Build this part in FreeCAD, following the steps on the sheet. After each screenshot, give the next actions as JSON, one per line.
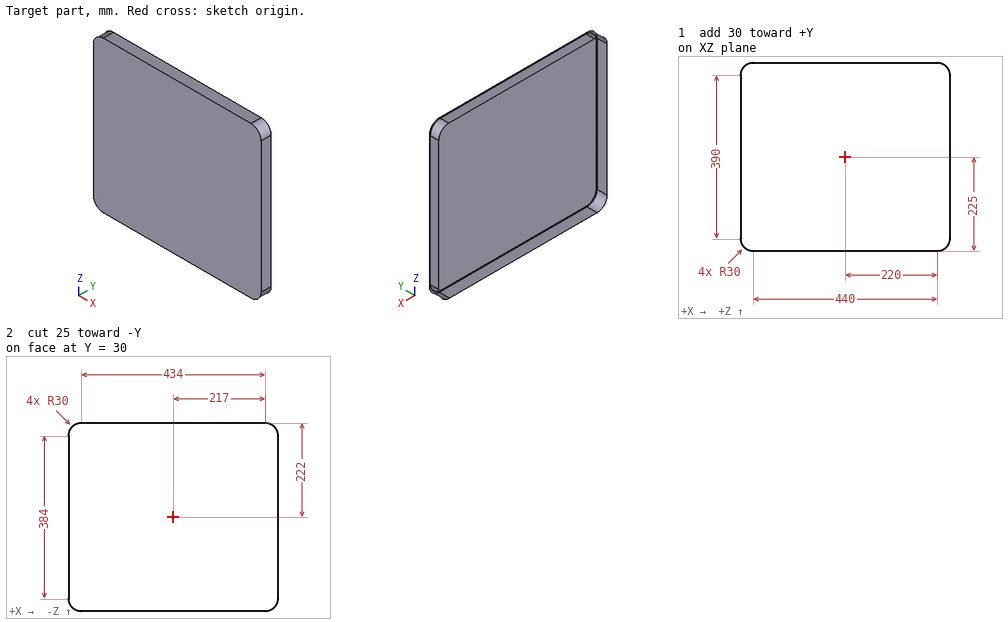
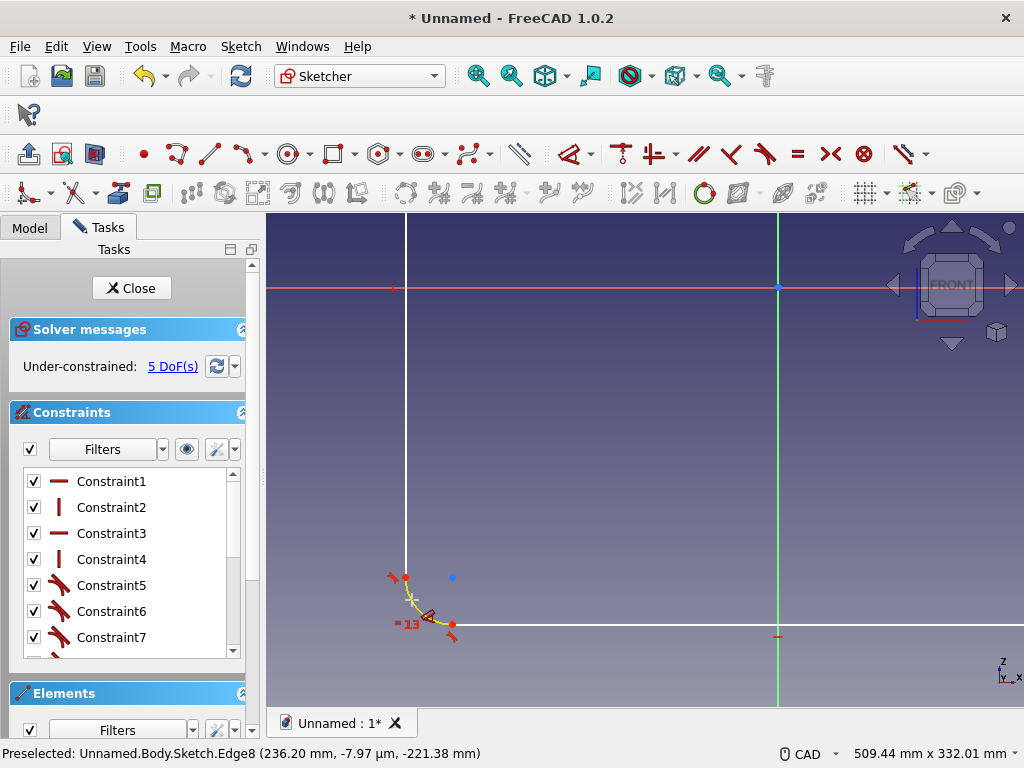
{"action": "left_click", "coordinate": [411, 599]}
{"action": "left_click", "coordinate": [382, 614]}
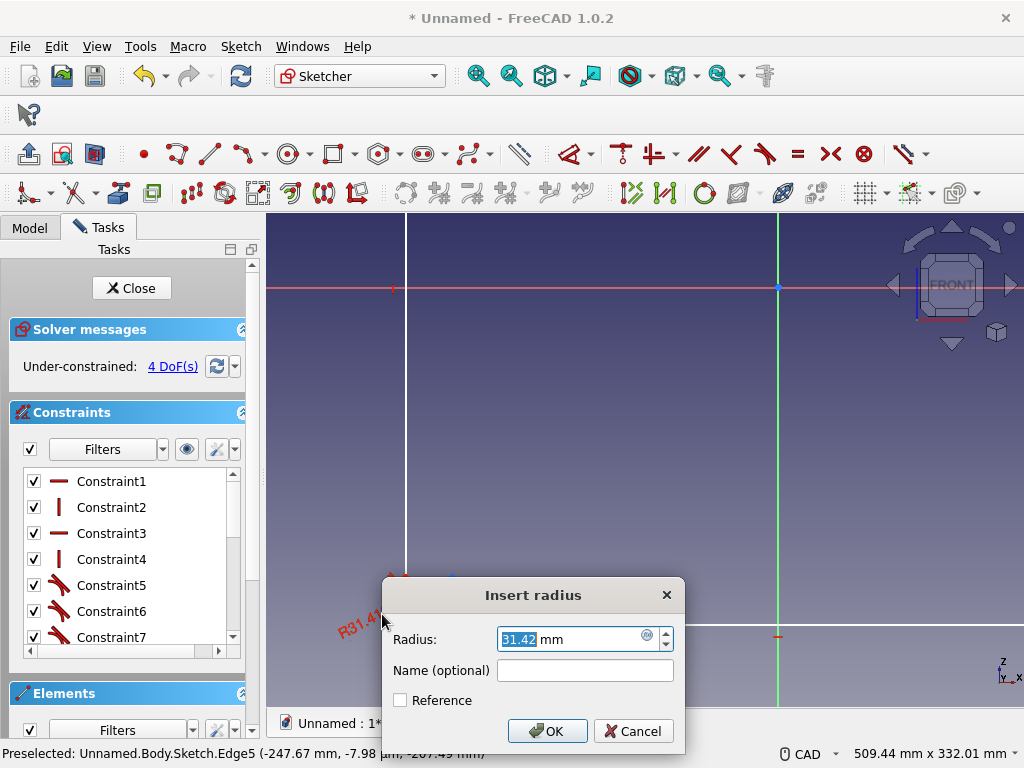
{"action": "type", "text": "30"}
{"action": "key", "text": "Return"}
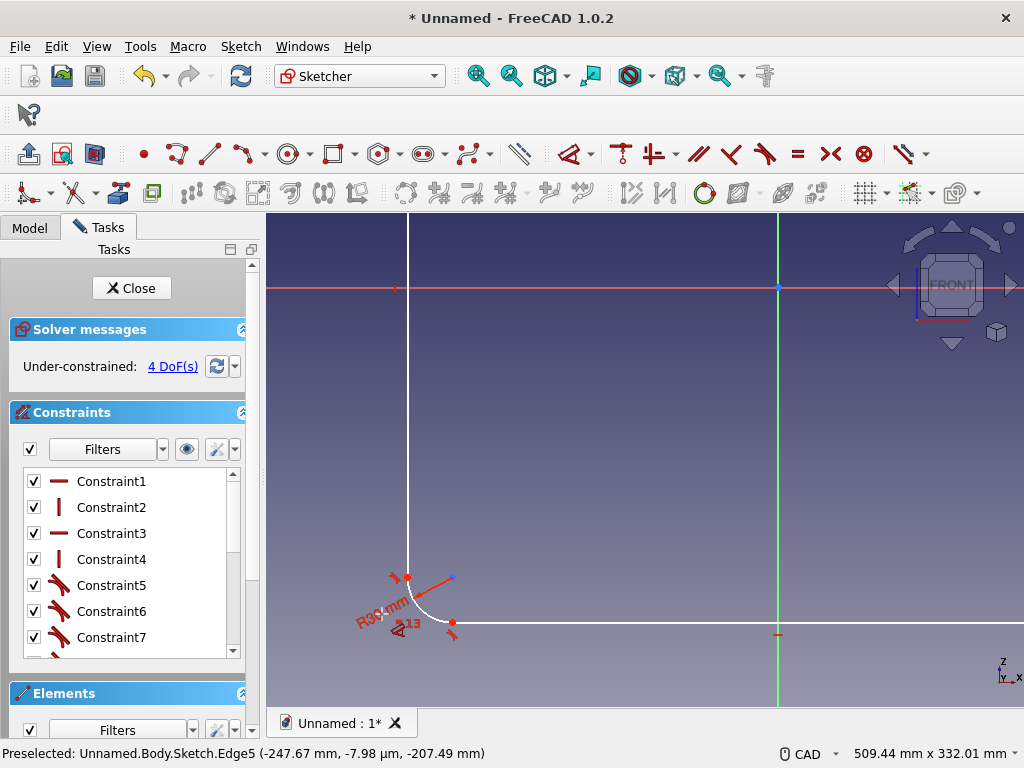
{"action": "left_click", "coordinate": [648, 623]}
{"action": "left_click", "coordinate": [656, 657]}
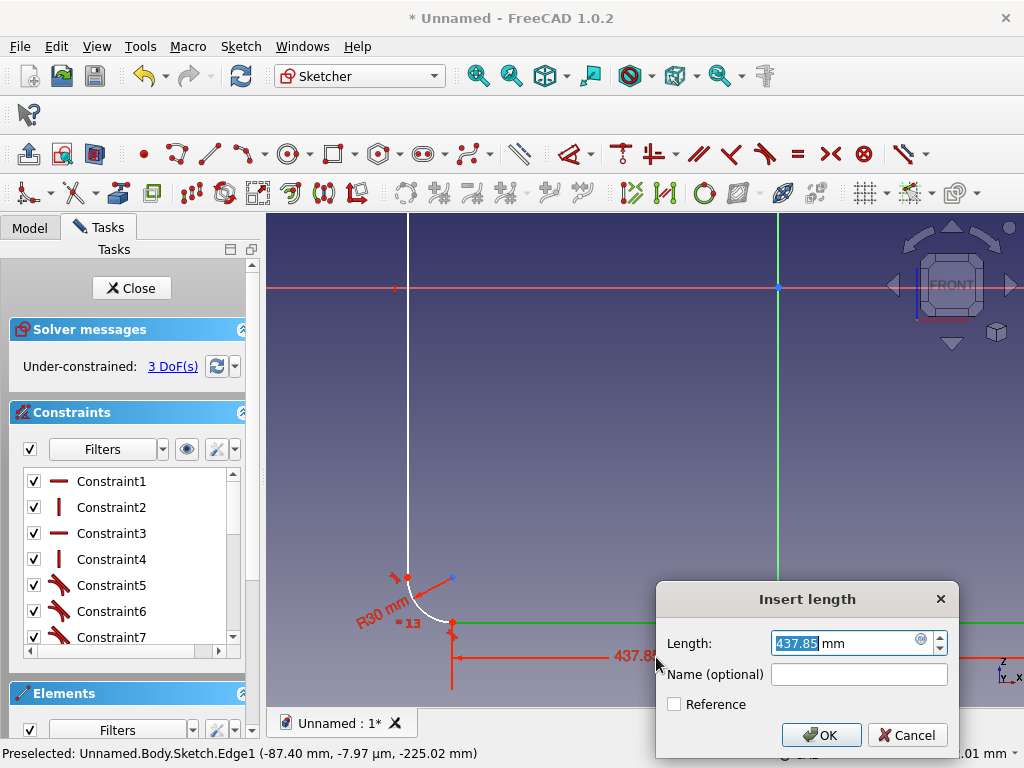
{"action": "type", "text": "440"}
{"action": "key", "text": "Return"}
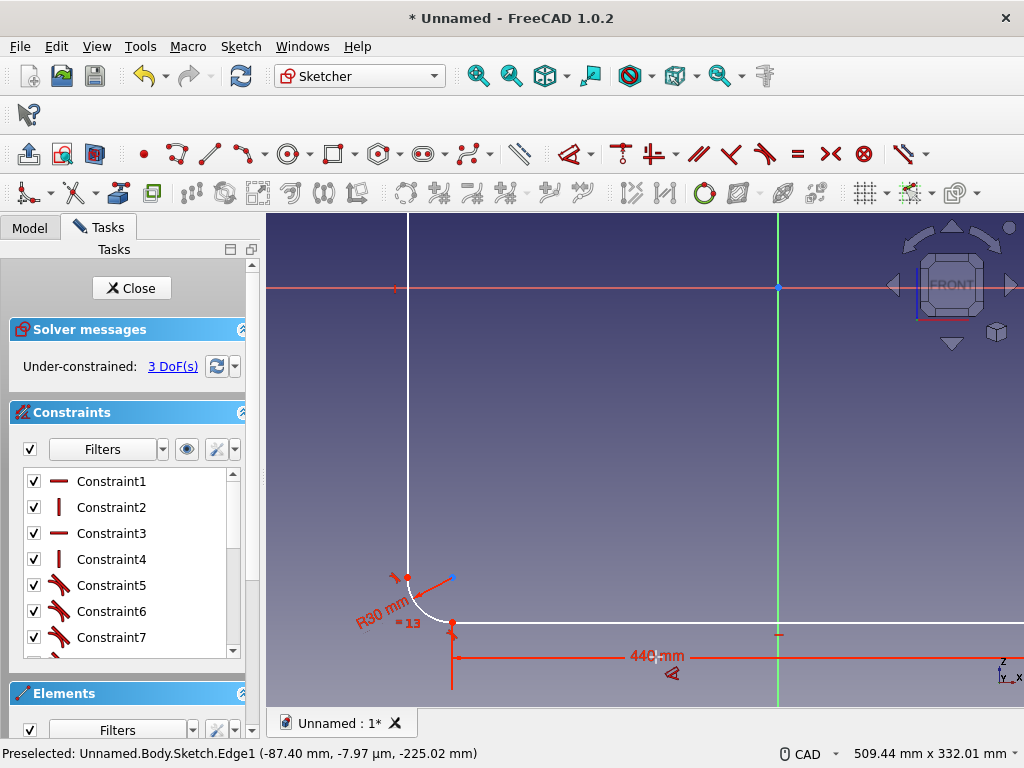
{"action": "left_click", "coordinate": [408, 404]}
{"action": "left_click", "coordinate": [374, 409]}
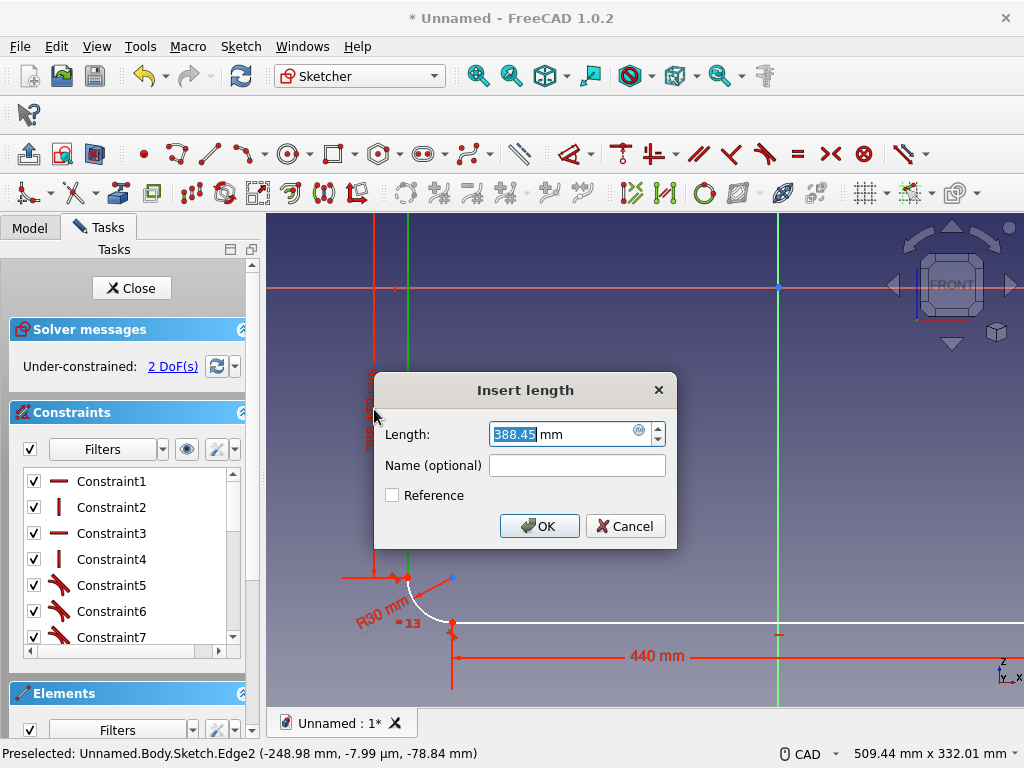
{"action": "type", "text": "390"}
{"action": "key", "text": "Return"}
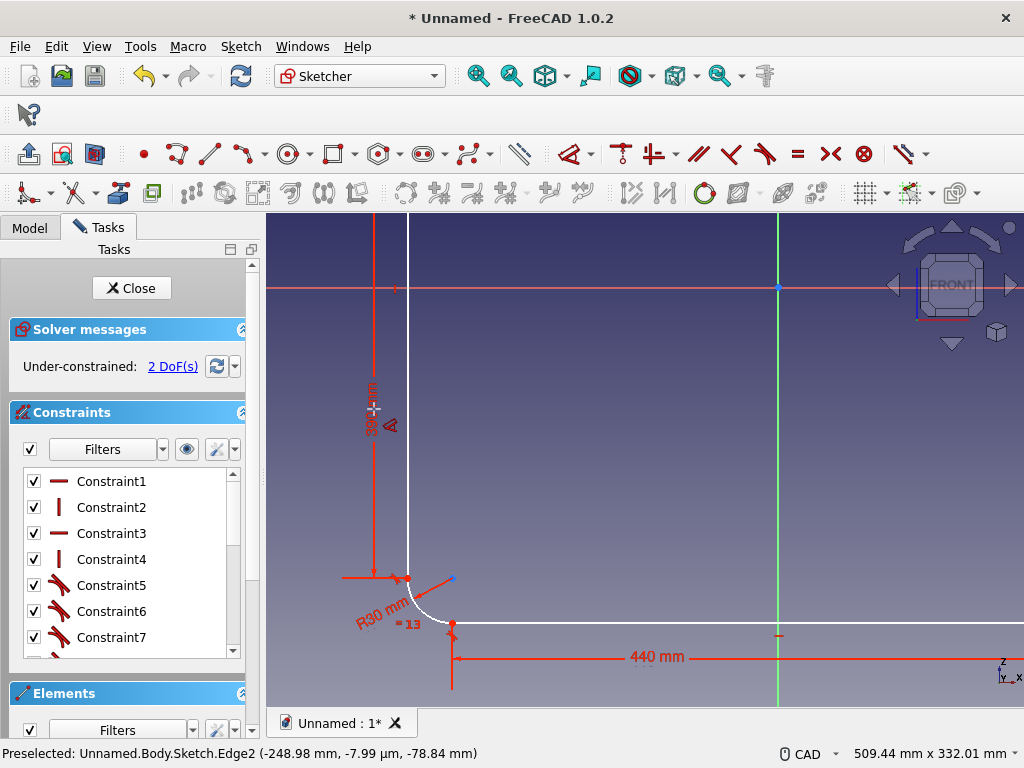
{"action": "scroll", "coordinate": [412, 601], "scroll_direction": "down", "scroll_amount": 4}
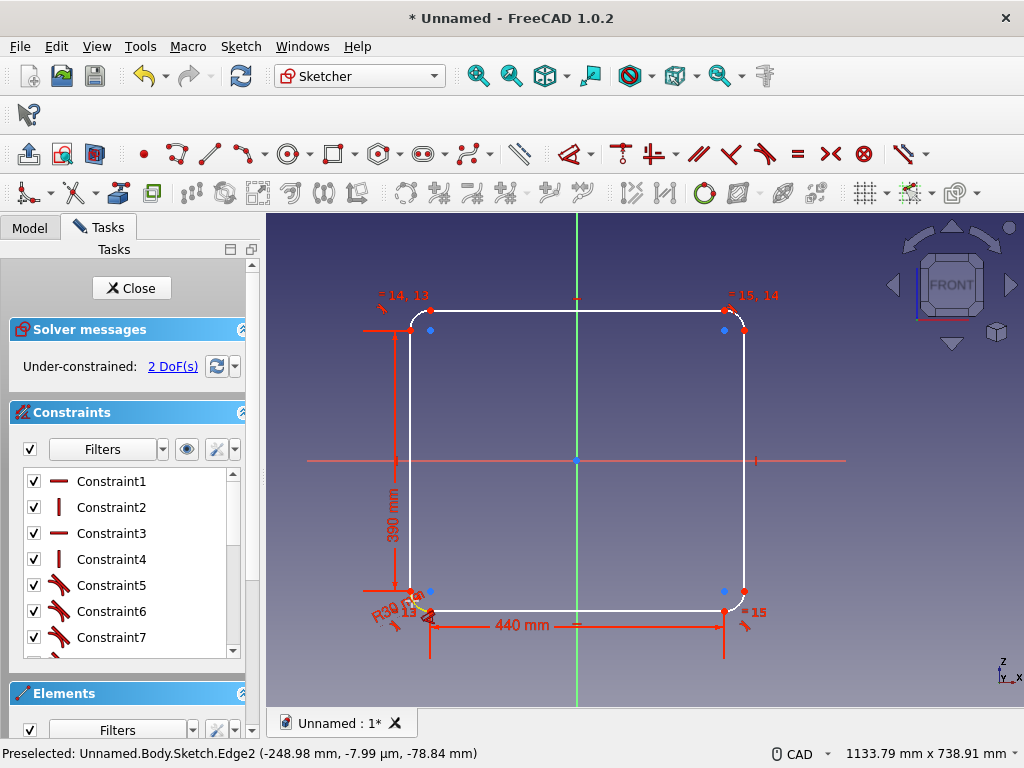
{"action": "left_click", "coordinate": [724, 611]}
{"action": "left_click", "coordinate": [650, 645]}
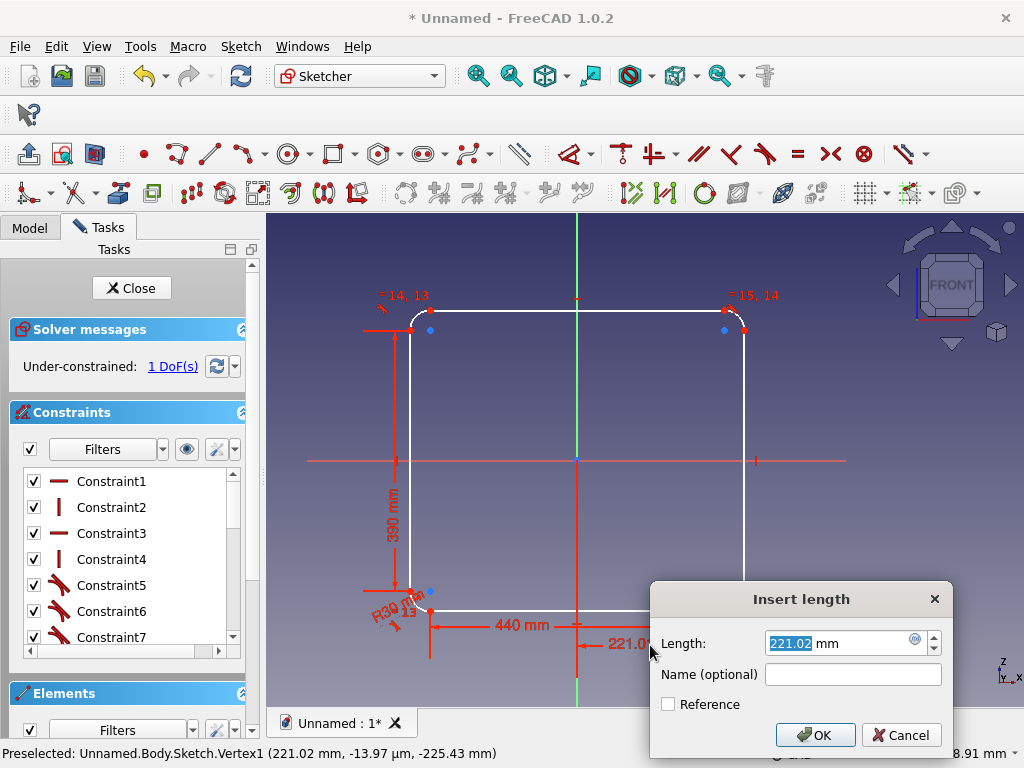
{"action": "type", "text": "220"}
{"action": "key", "text": "Return"}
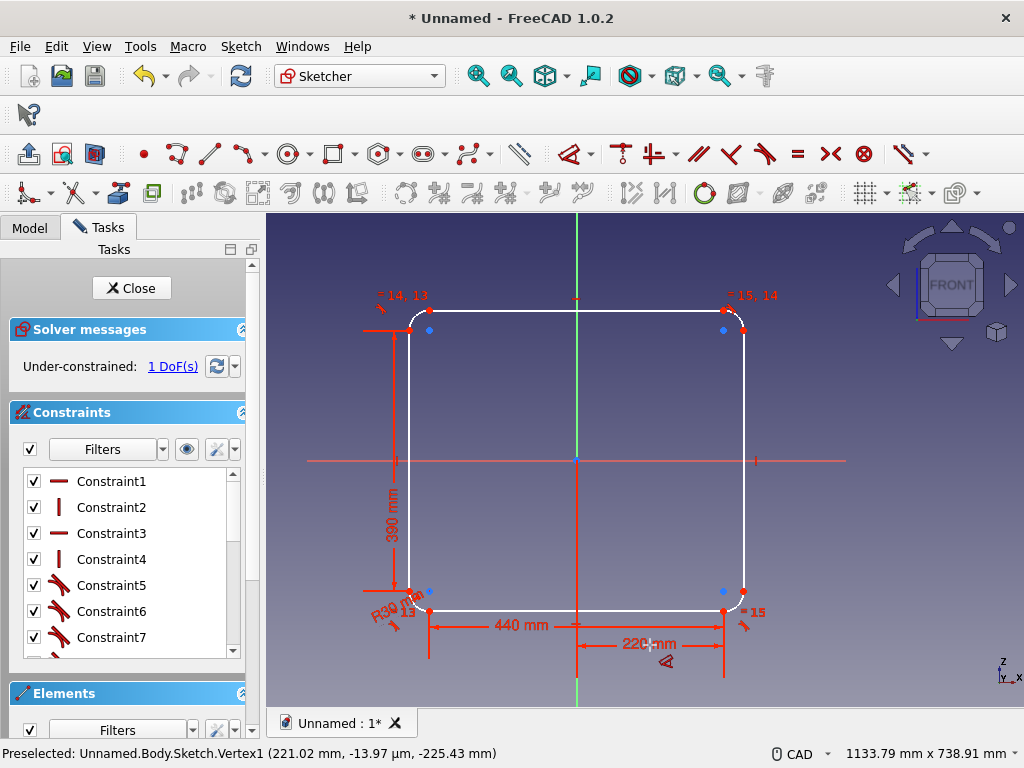
{"action": "left_click", "coordinate": [724, 611]}
{"action": "left_click", "coordinate": [758, 536]}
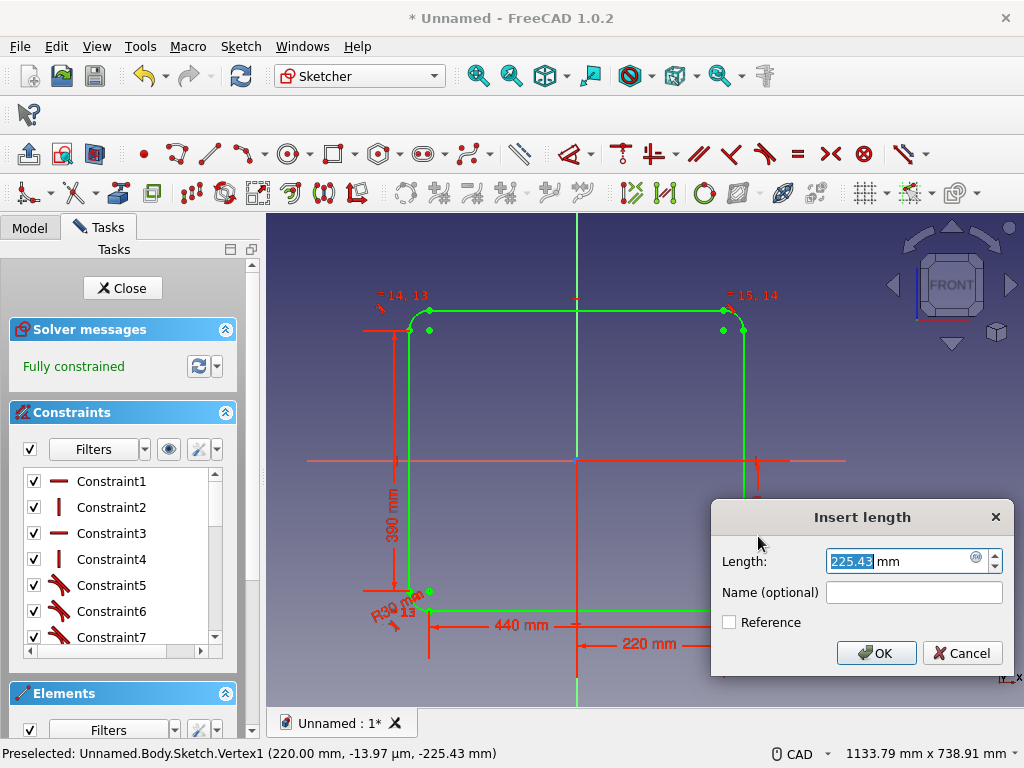
{"action": "type", "text": "225"}
{"action": "key", "text": "Return"}
{"action": "key", "text": "Escape"}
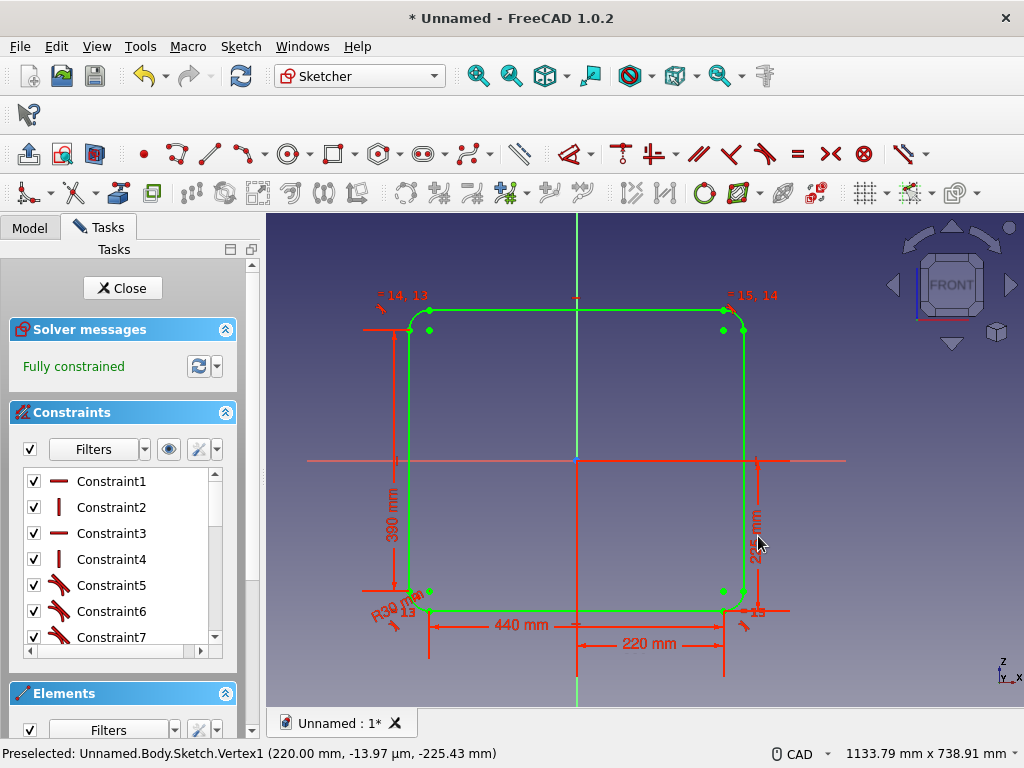
{"action": "left_click", "coordinate": [123, 288]}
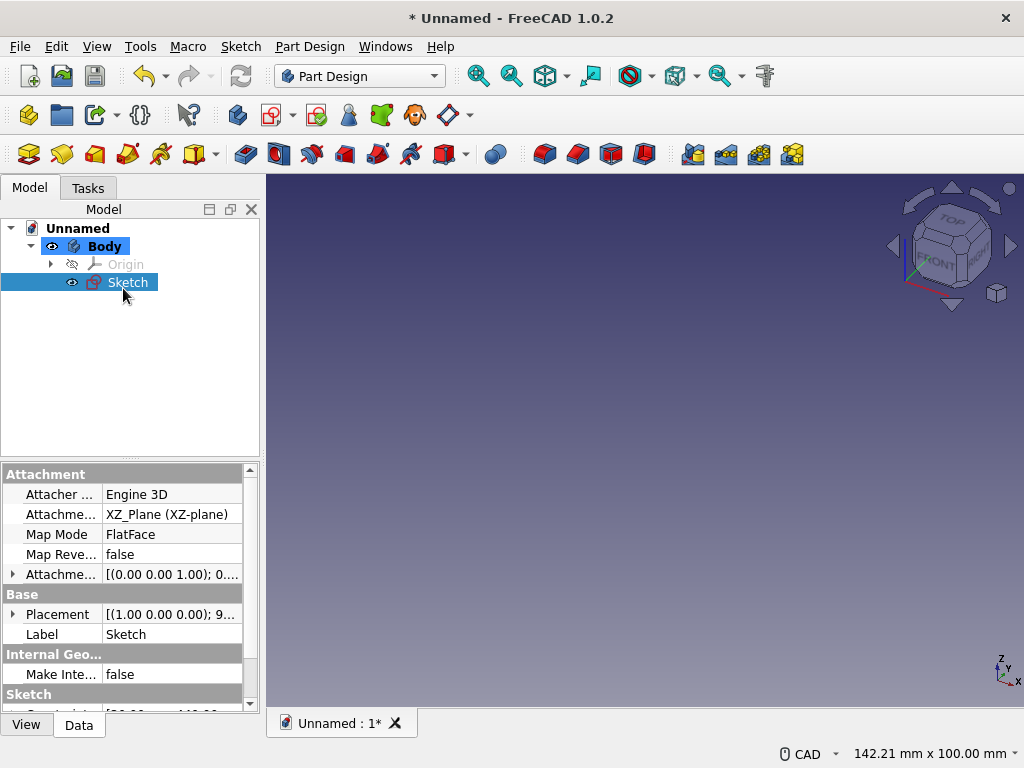
{"action": "left_click", "coordinate": [29, 154]}